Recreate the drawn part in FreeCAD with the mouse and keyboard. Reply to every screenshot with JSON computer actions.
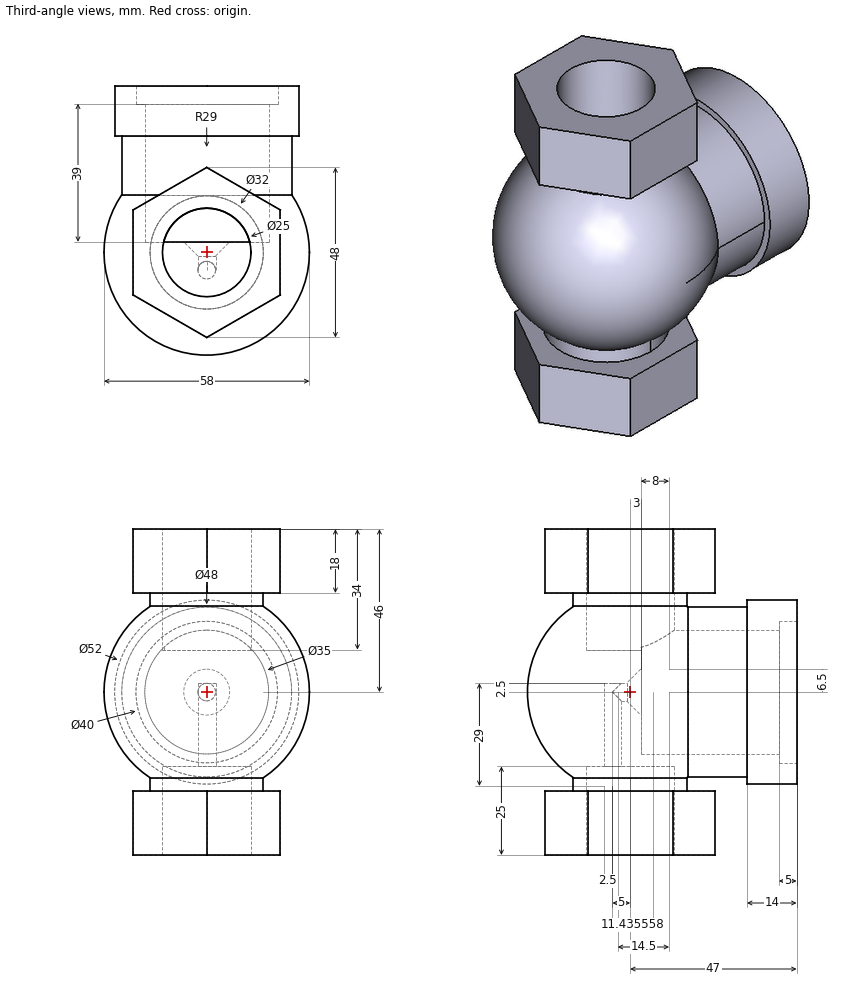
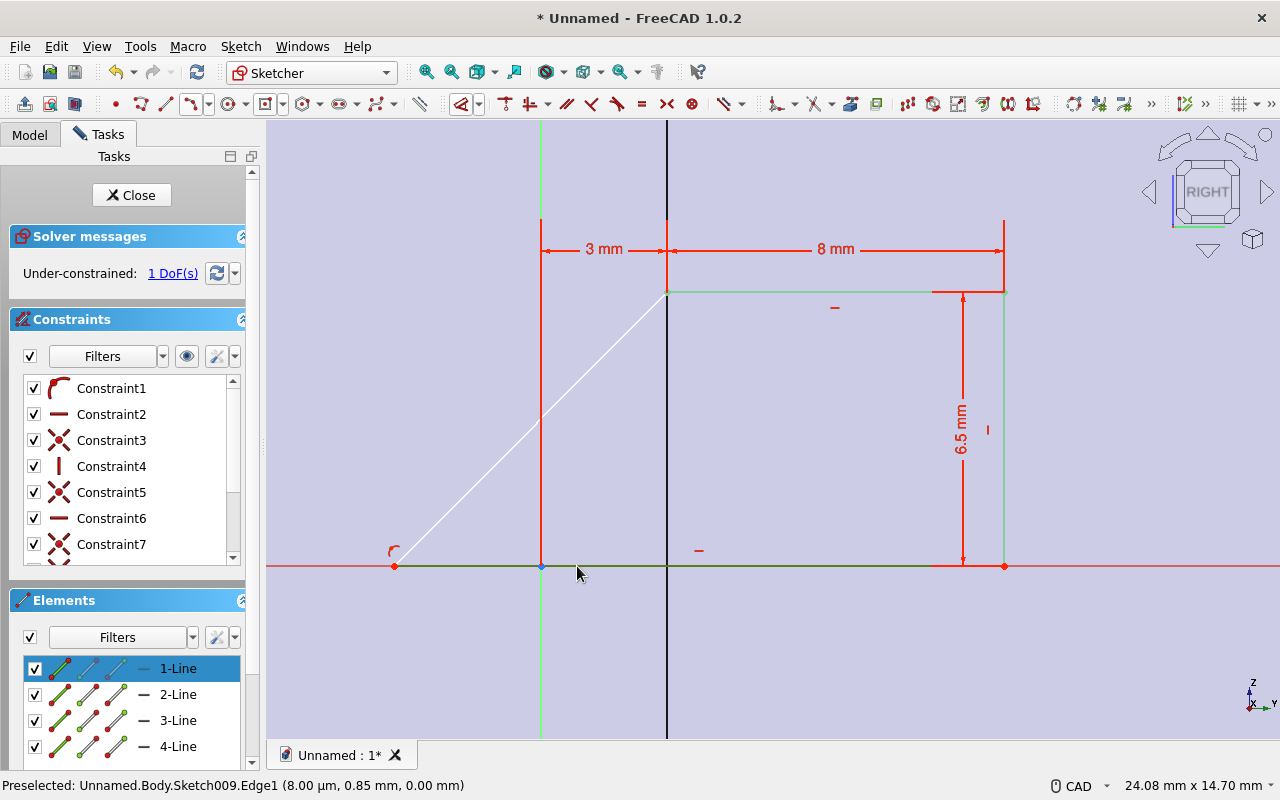
{"action": "key", "text": "l"}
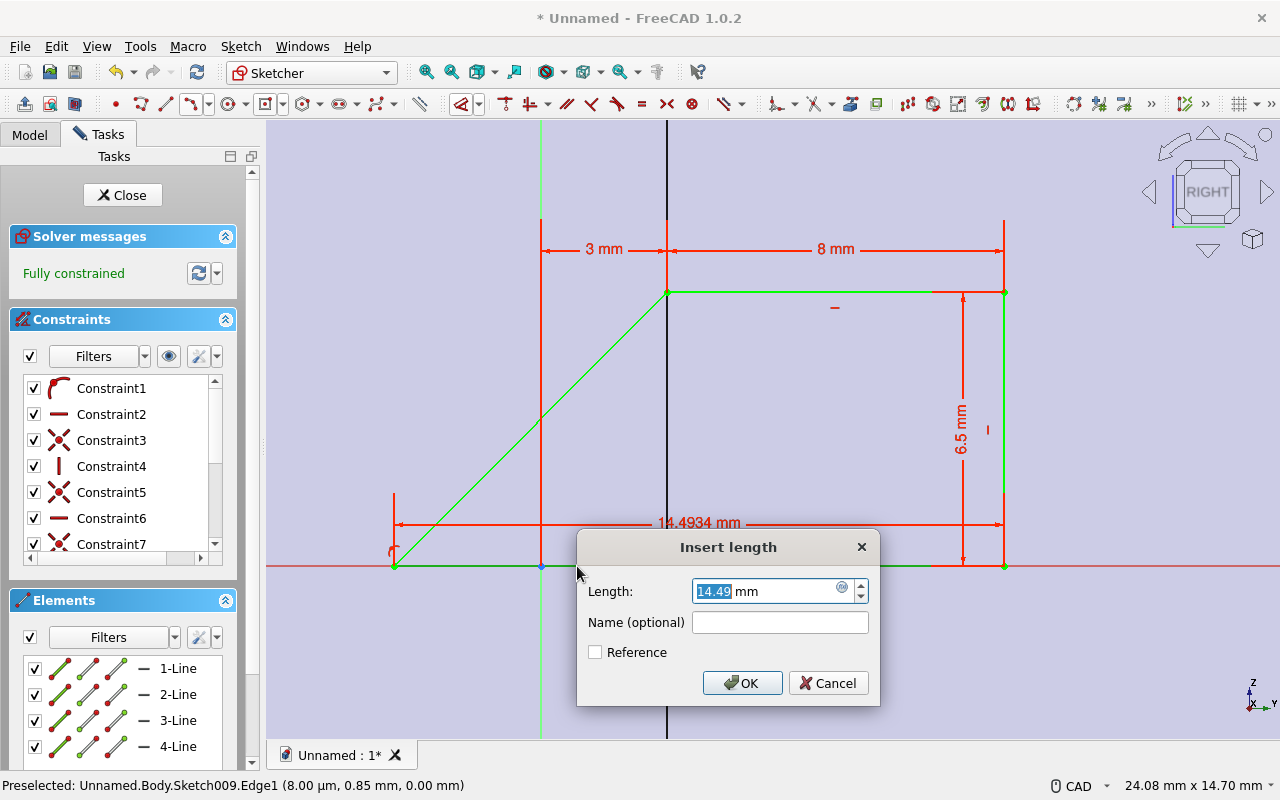
{"action": "type", "text": "14.5"}
{"action": "key", "text": "Return"}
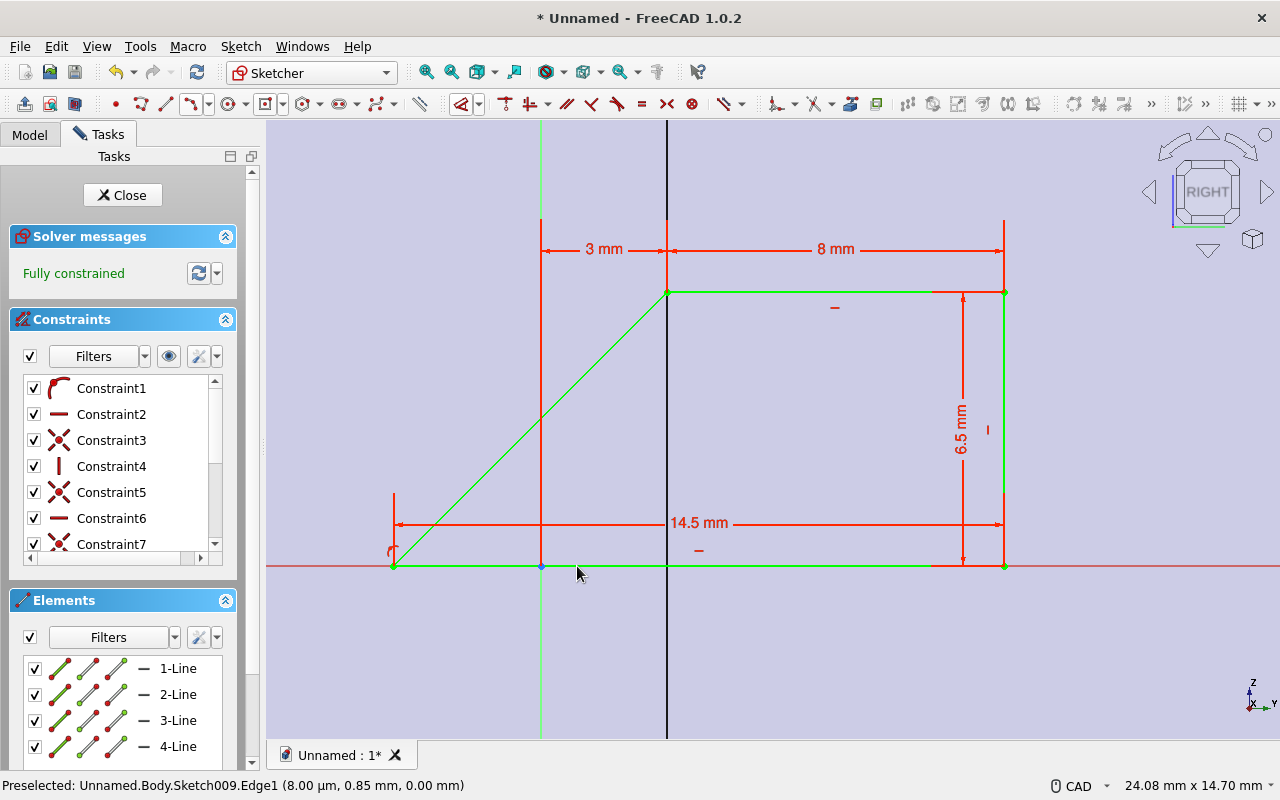
{"action": "left_click", "coordinate": [123, 195]}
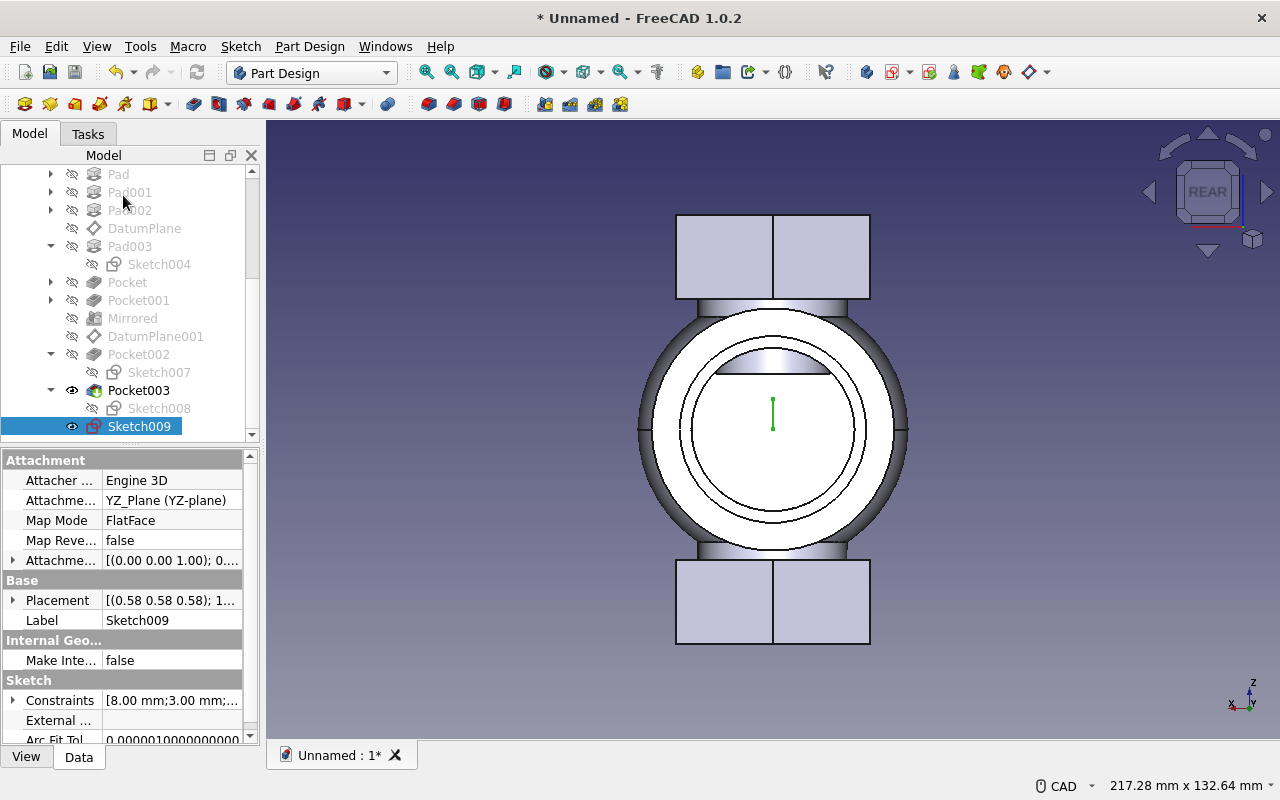
{"action": "left_click", "coordinate": [244, 104]}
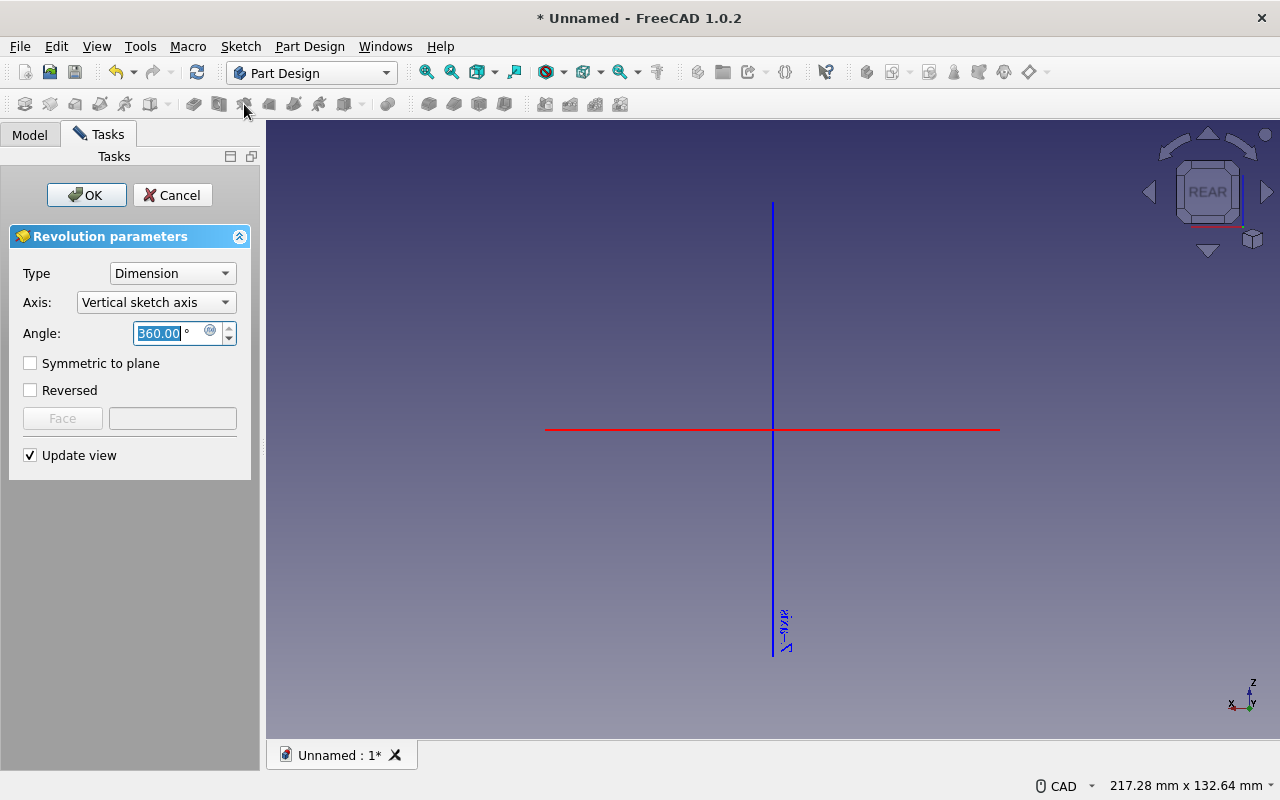
{"action": "left_click", "coordinate": [157, 302]}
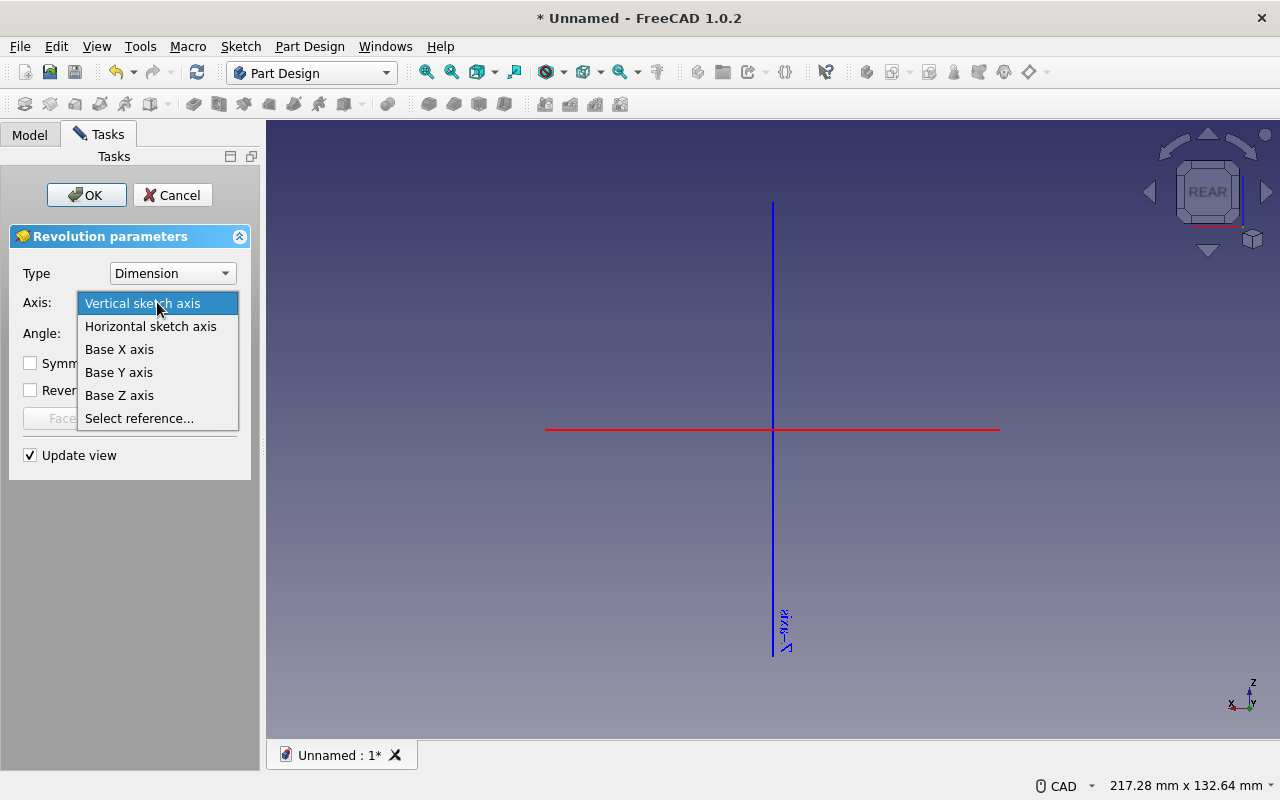
{"action": "left_click", "coordinate": [156, 326]}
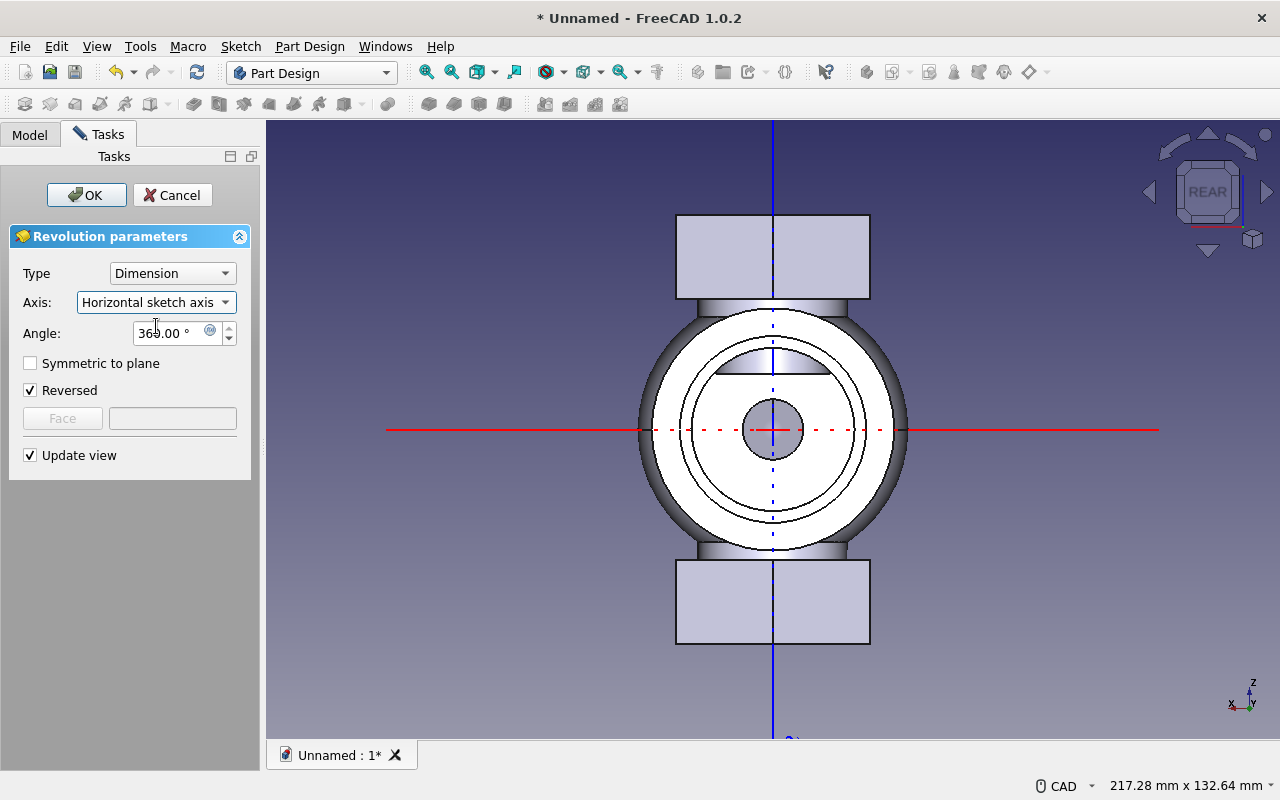
{"action": "left_click", "coordinate": [87, 195]}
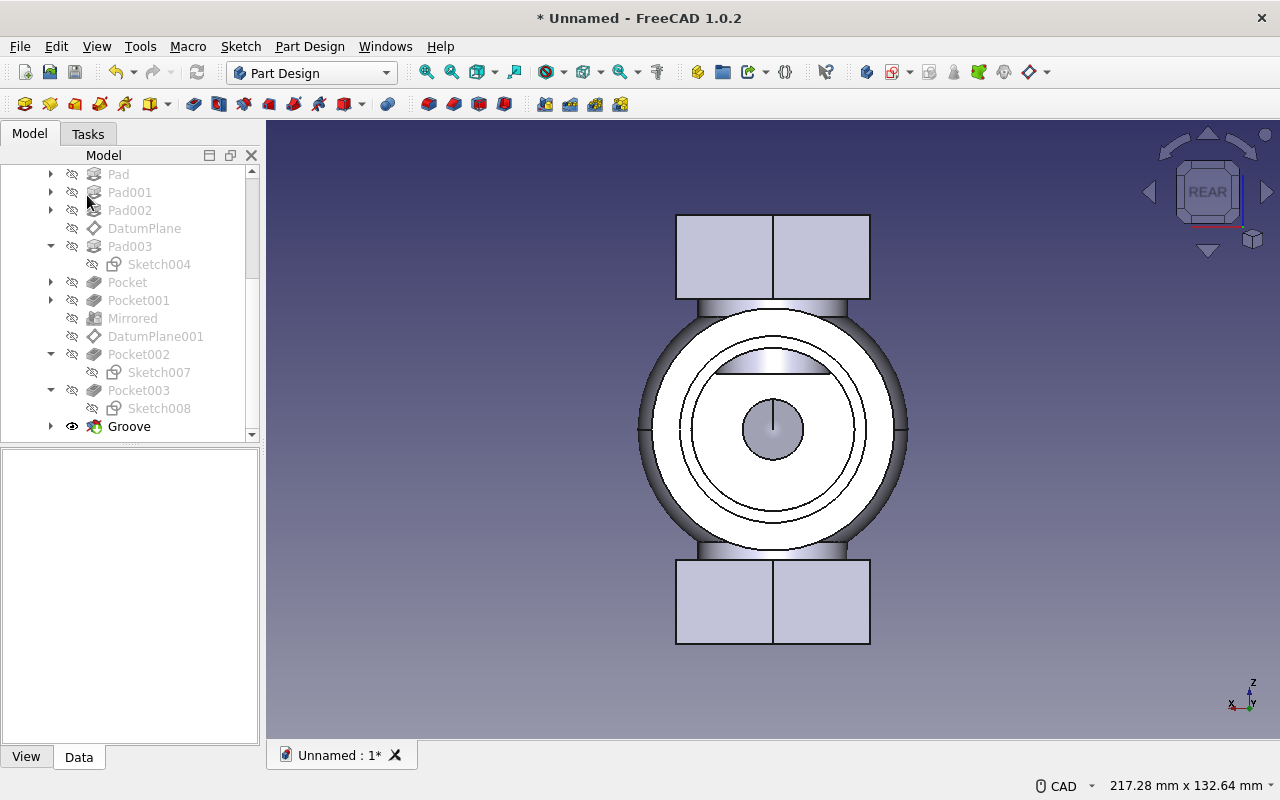
{"action": "left_click", "coordinate": [892, 72]}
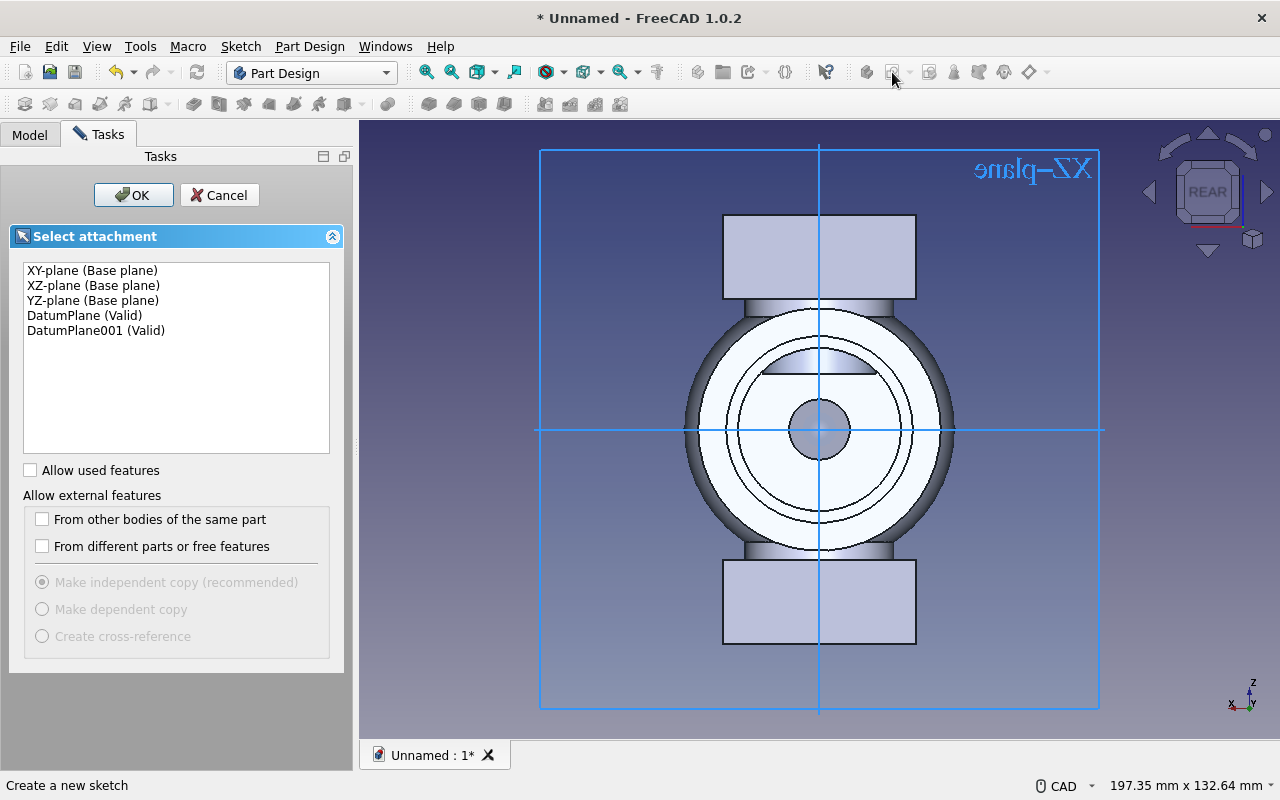
{"action": "left_click", "coordinate": [84, 300]}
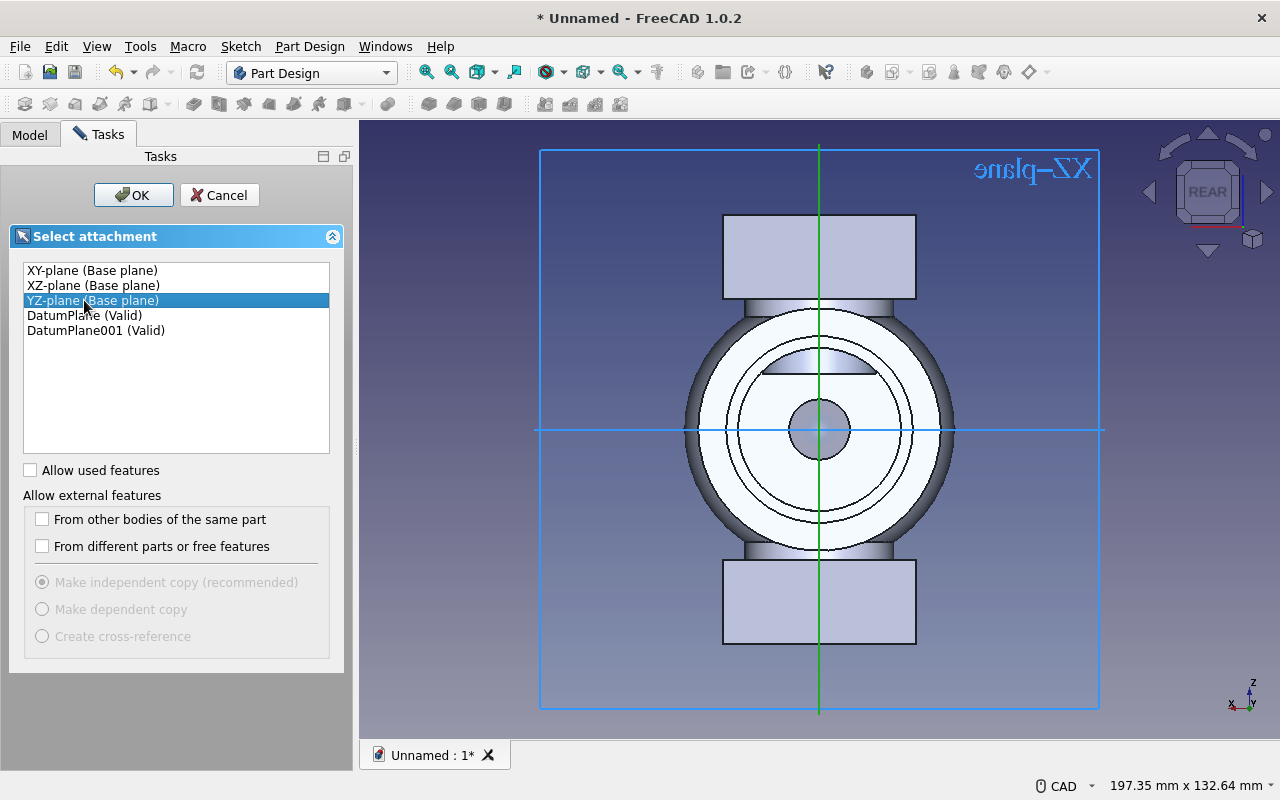
{"action": "left_click", "coordinate": [134, 195]}